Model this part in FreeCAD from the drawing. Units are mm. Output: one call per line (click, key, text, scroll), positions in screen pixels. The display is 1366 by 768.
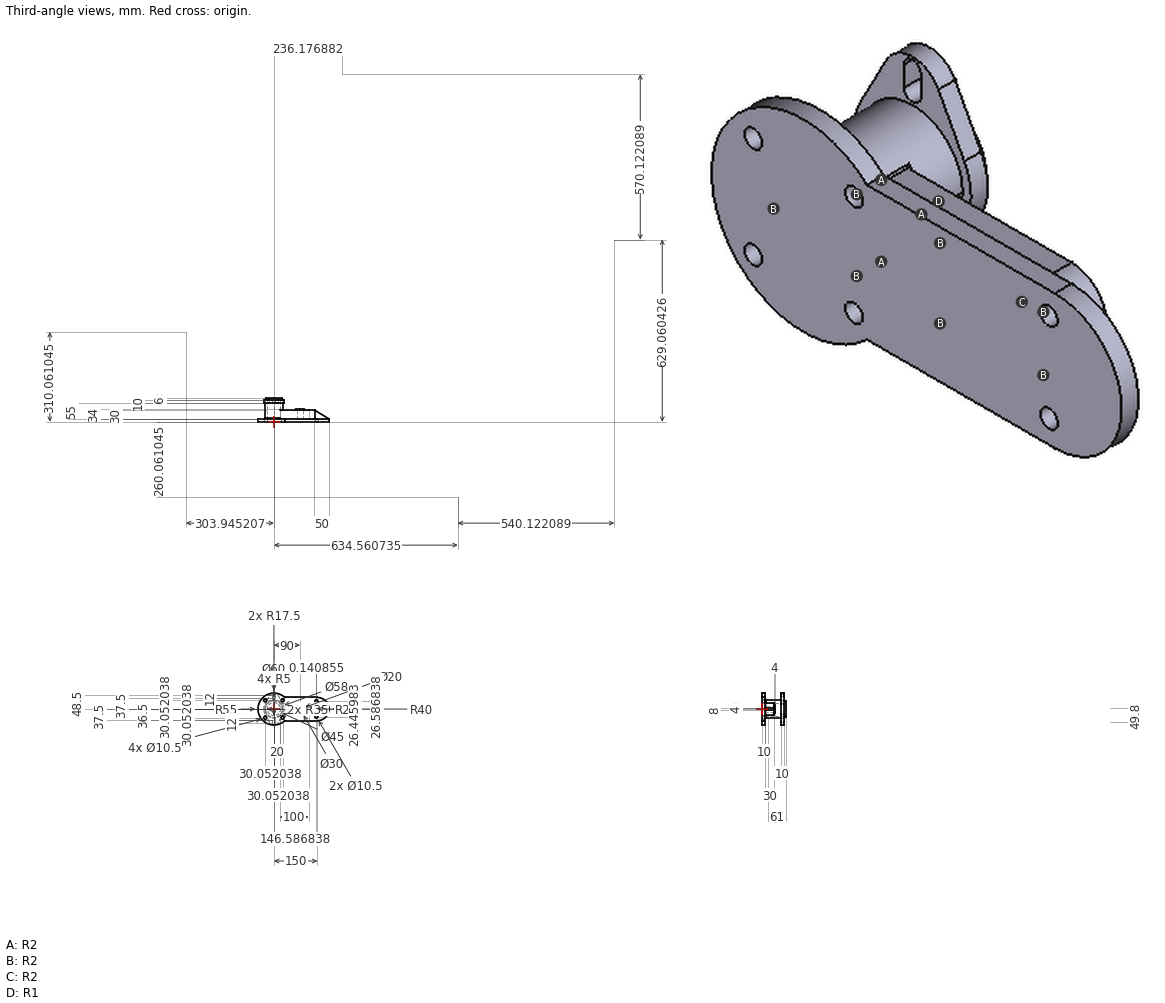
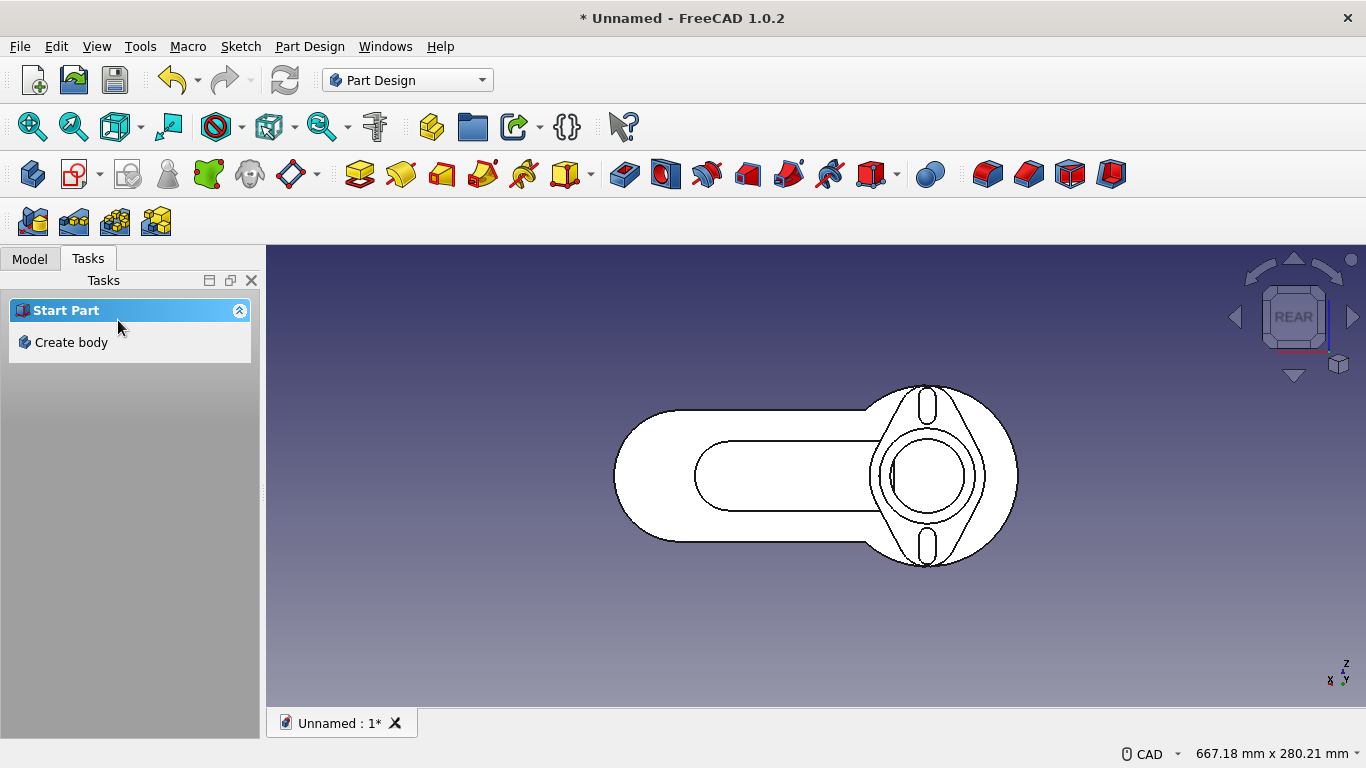
key(v)
key(f)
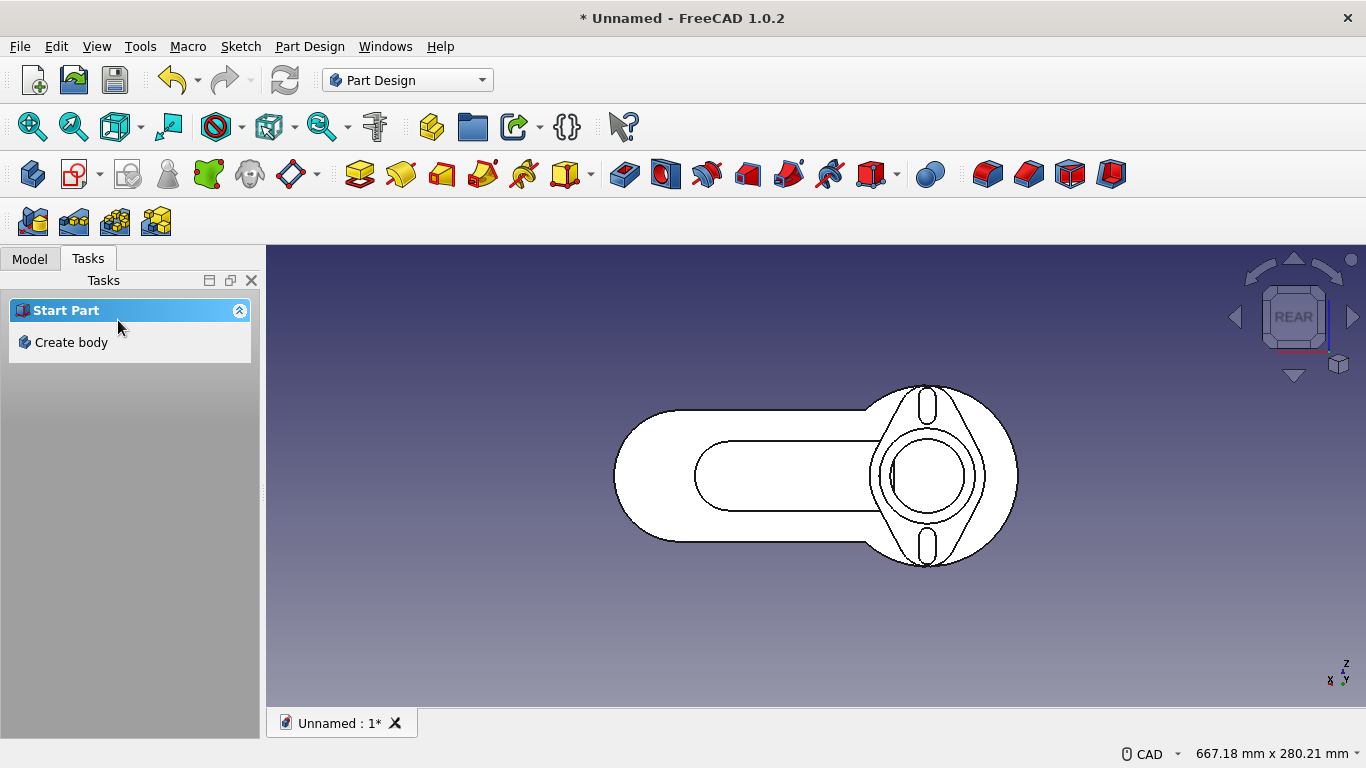
click(737, 475)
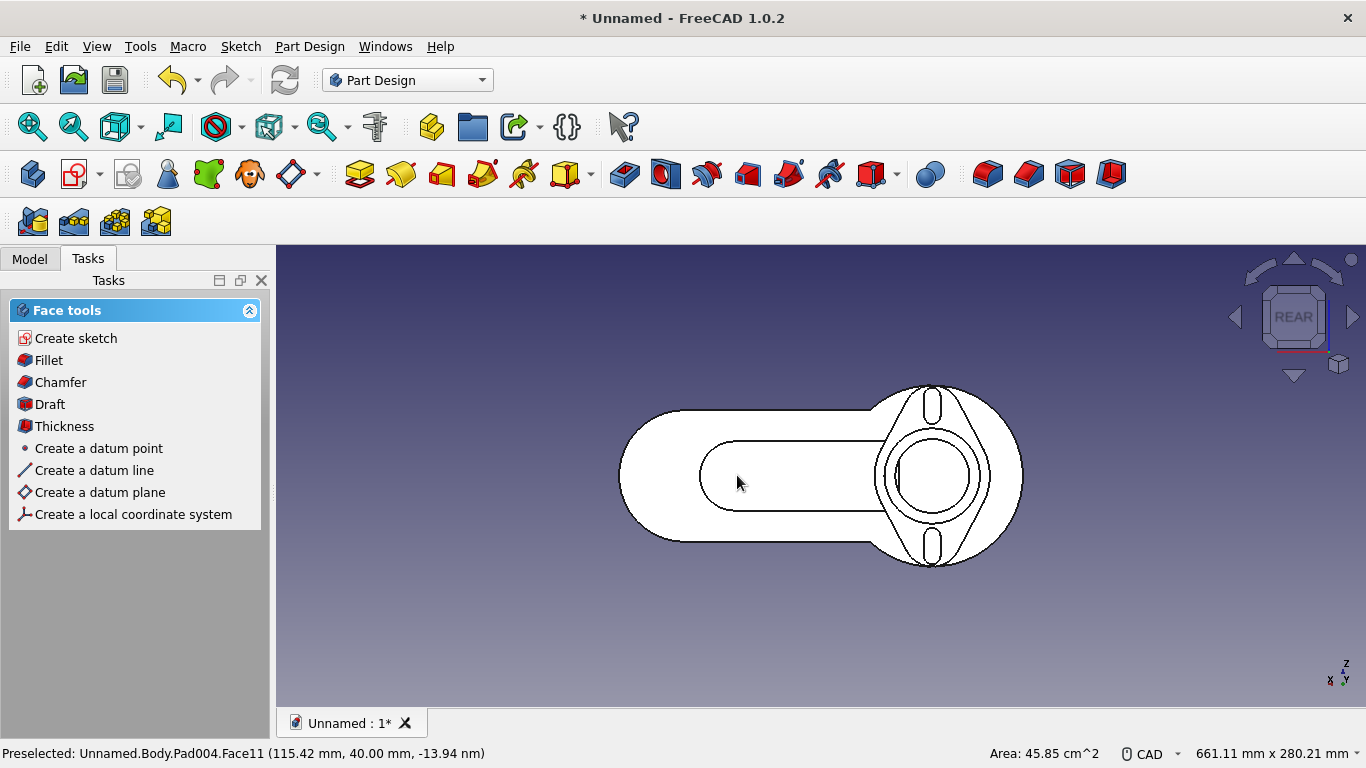
click(74, 174)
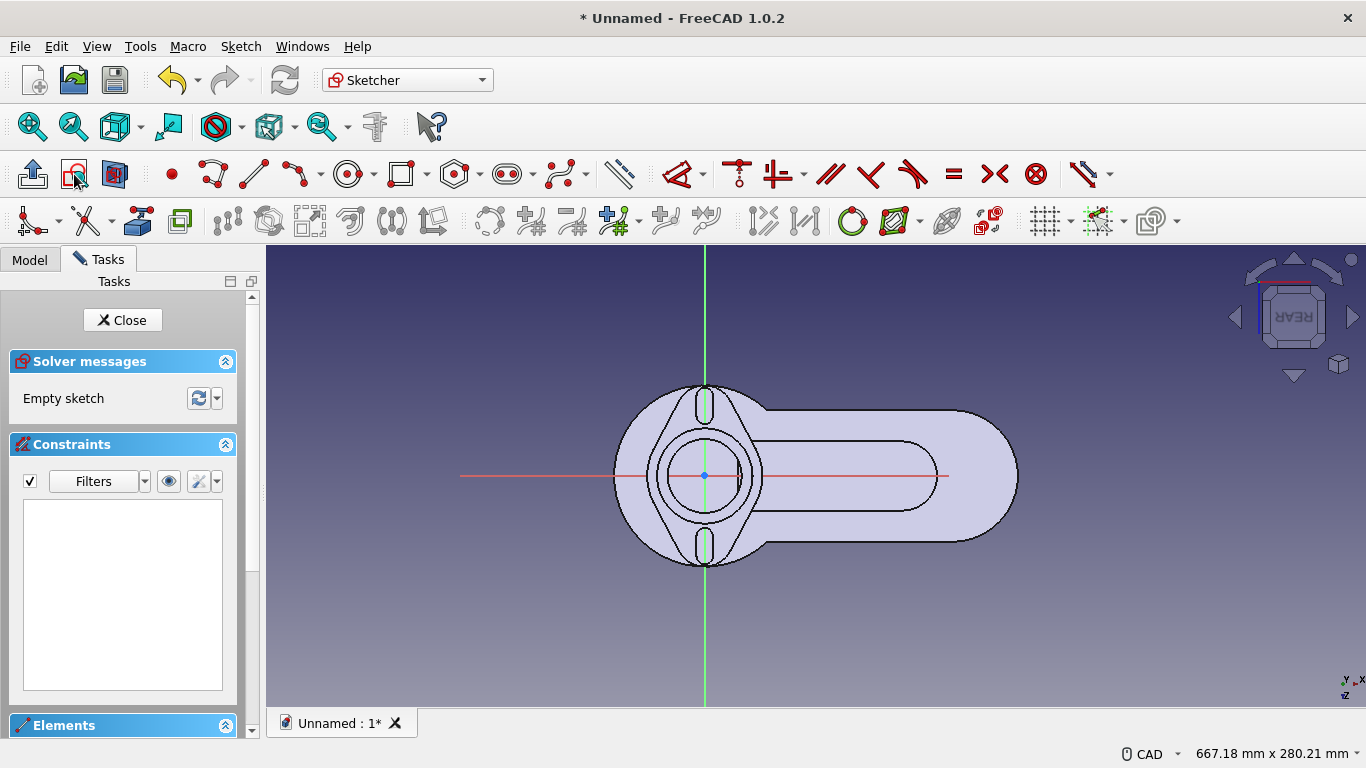
key(q)
key(s)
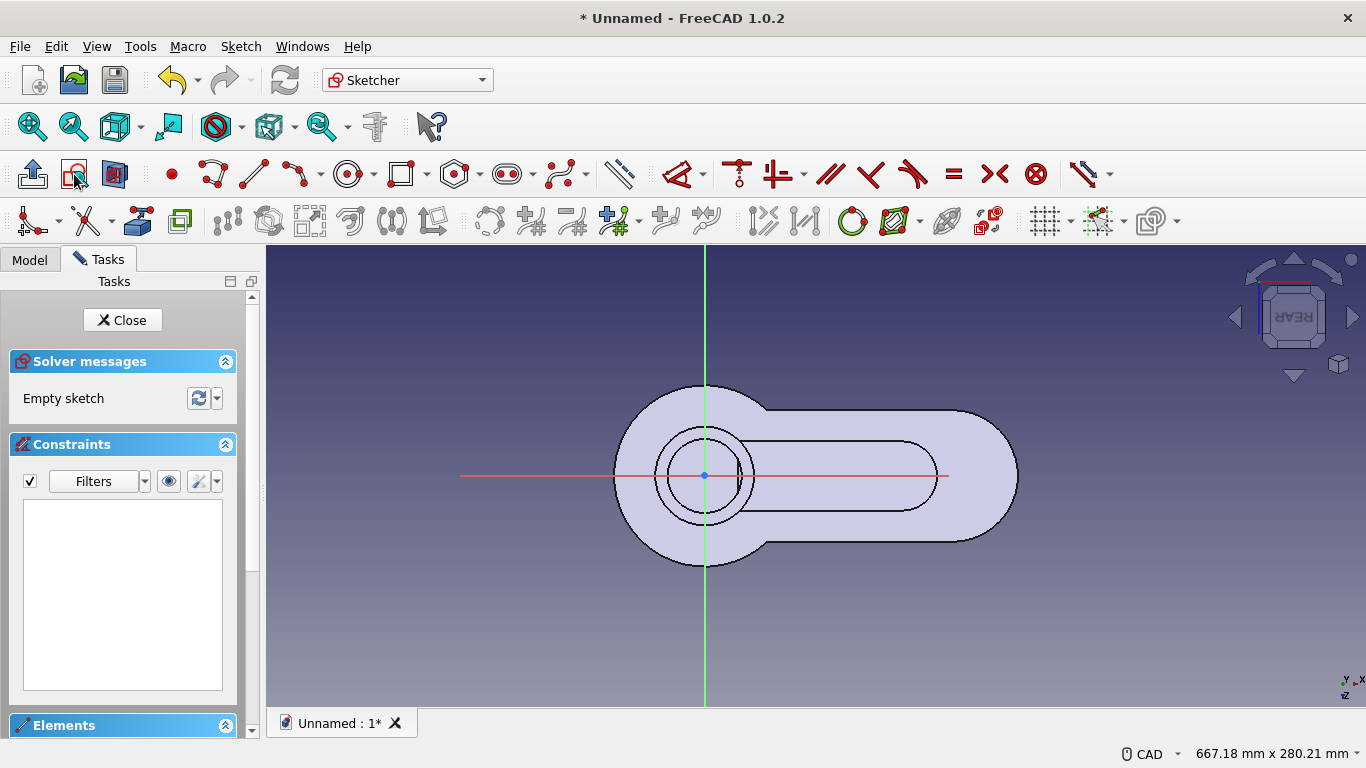
scroll(691, 476, up, 7)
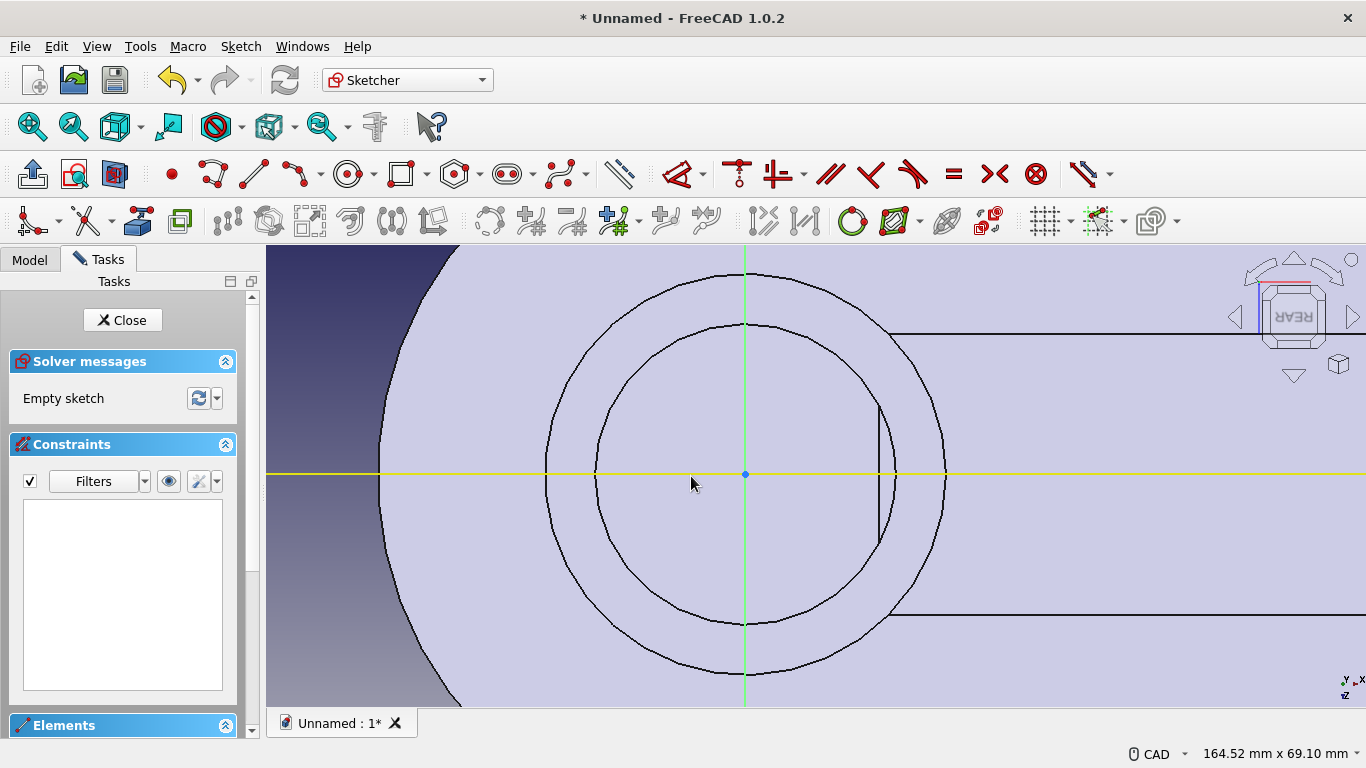
key(g)
key(c)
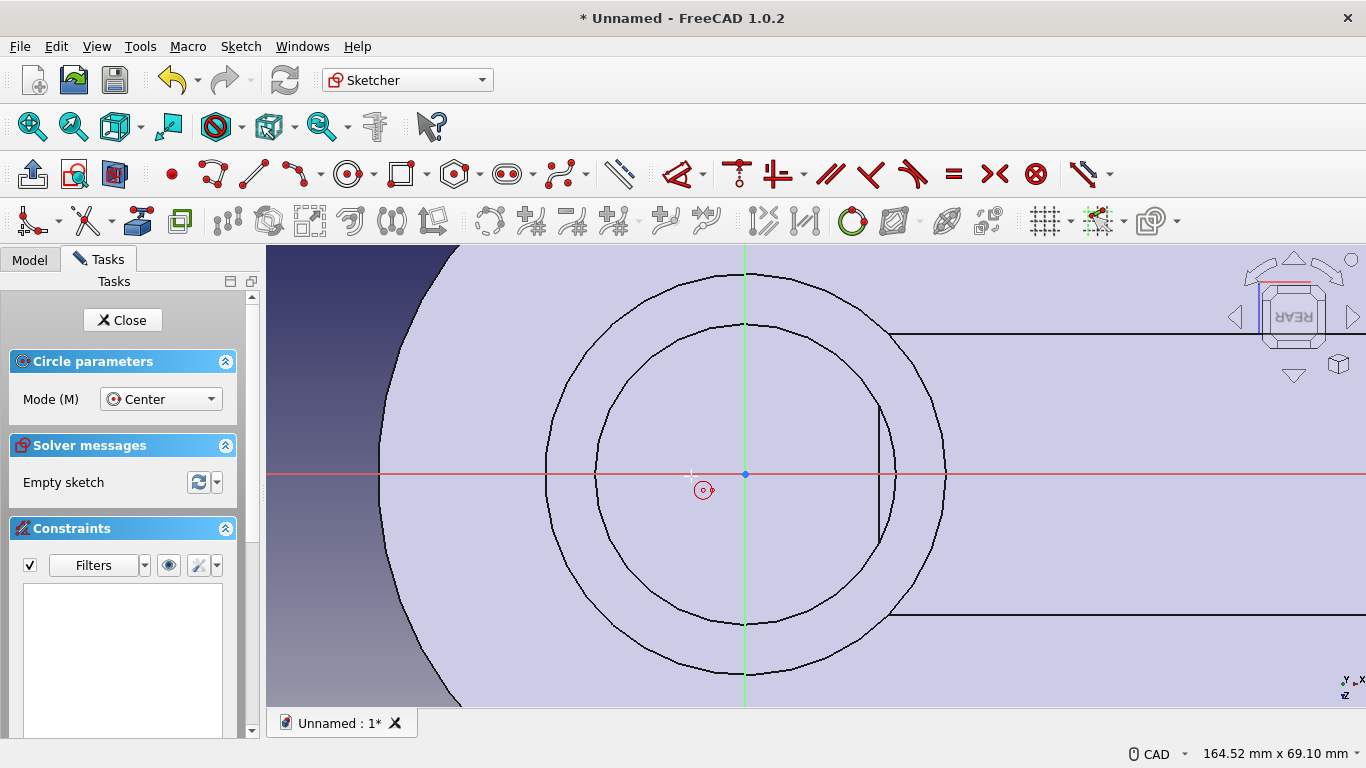
click(745, 474)
click(852, 368)
key(Escape)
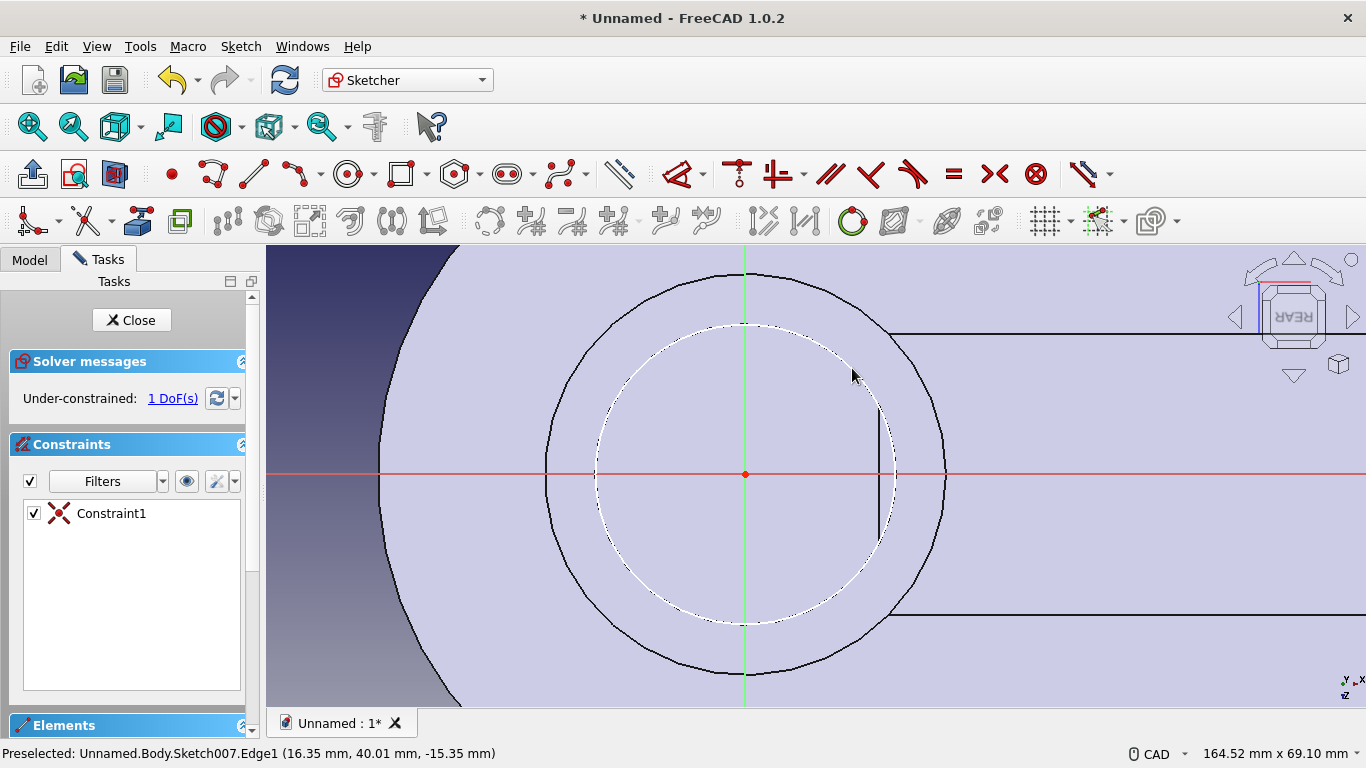
click(676, 174)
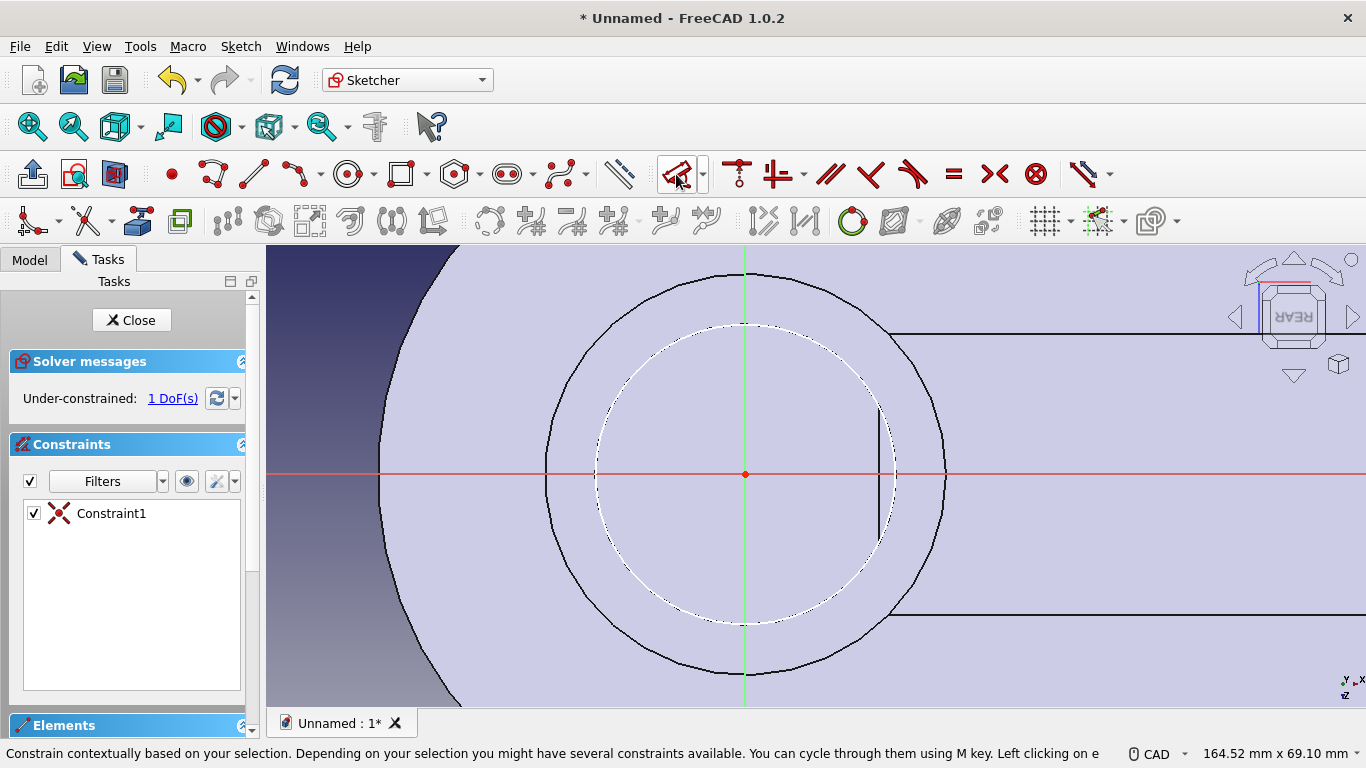
click(851, 368)
click(874, 345)